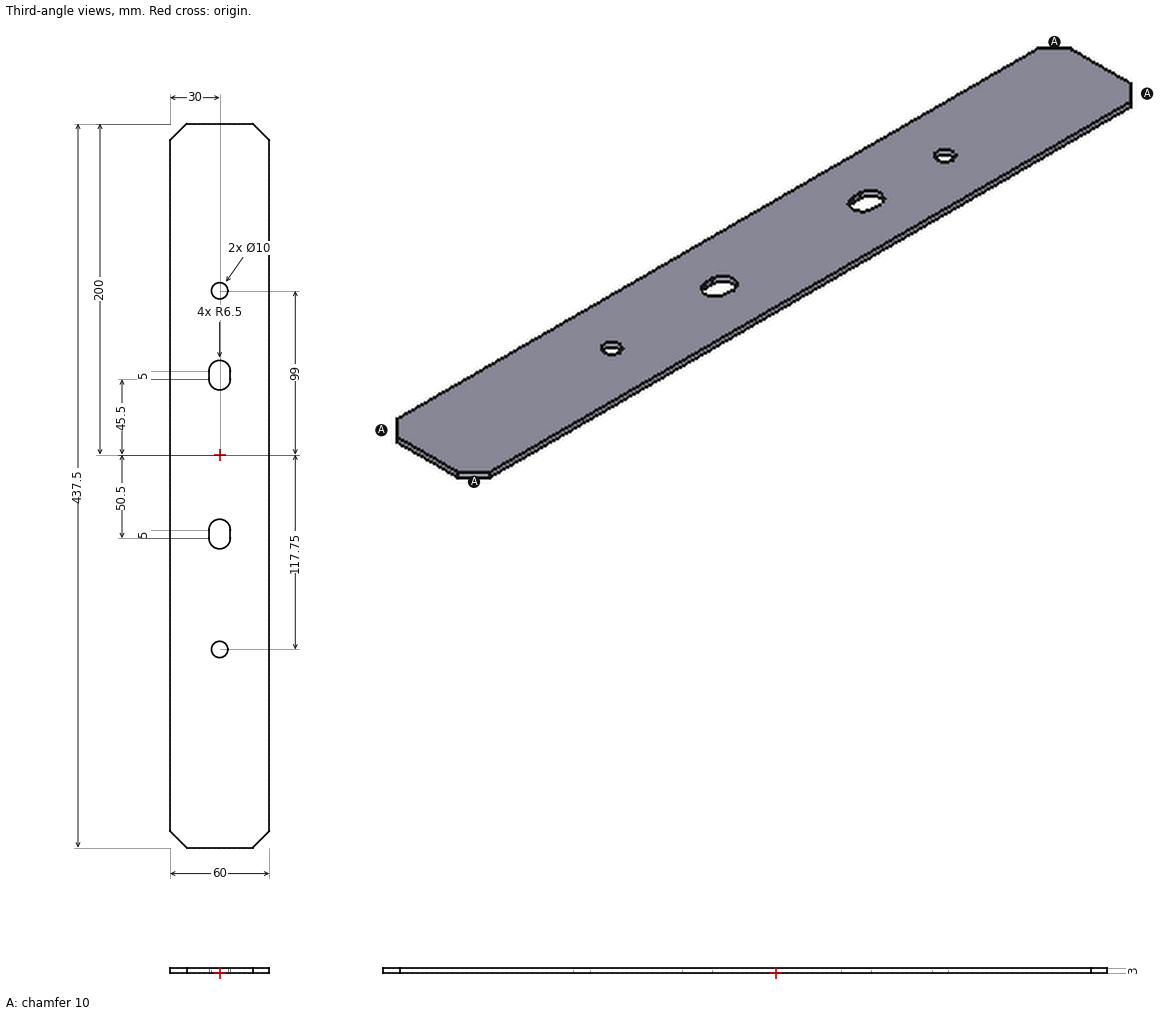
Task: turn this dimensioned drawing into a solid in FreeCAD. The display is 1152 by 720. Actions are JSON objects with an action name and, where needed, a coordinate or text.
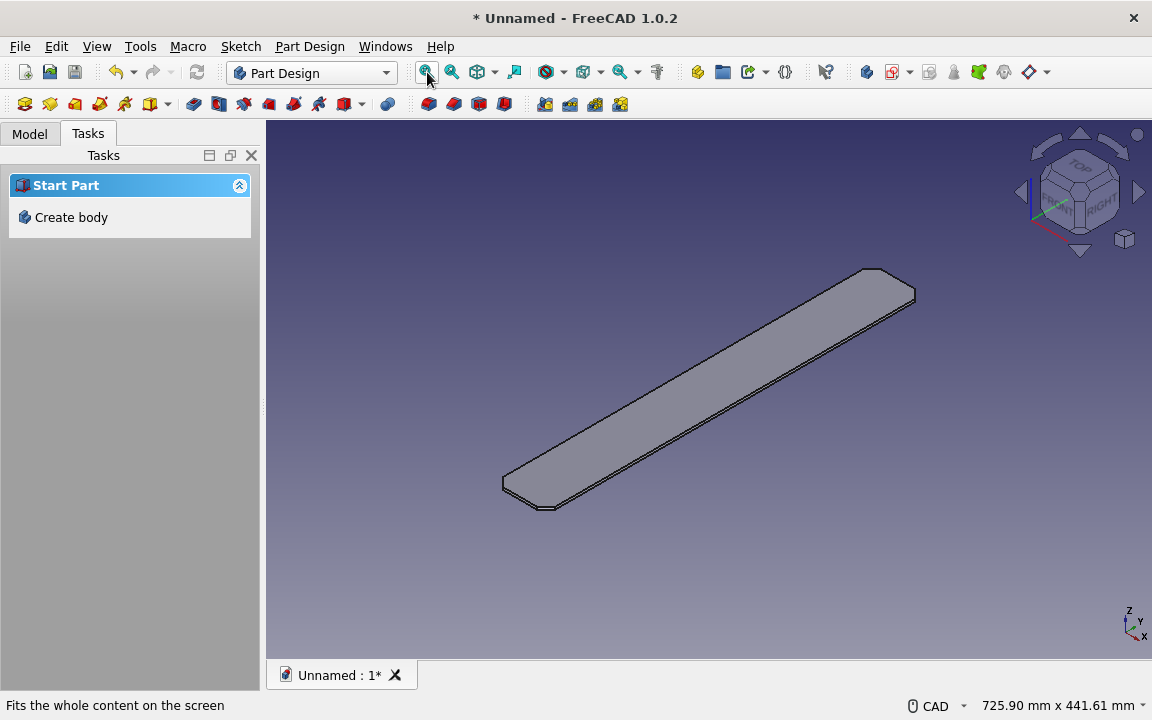
{"action": "left_click", "coordinate": [871, 294]}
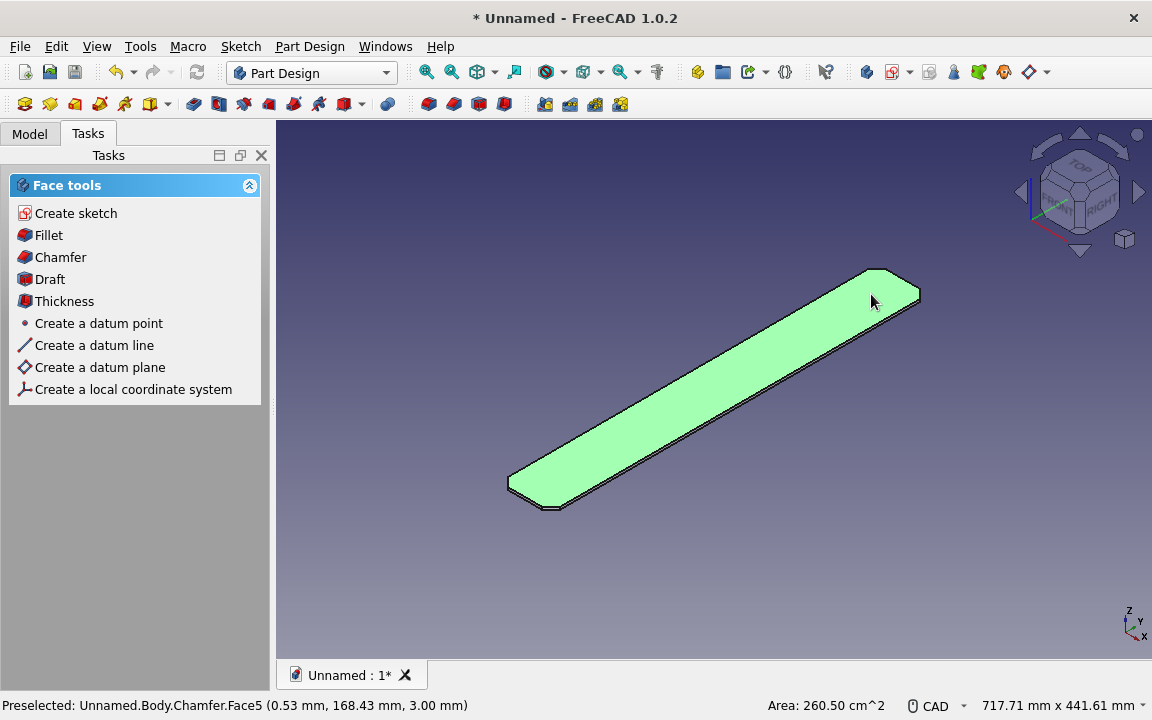
{"action": "left_click", "coordinate": [892, 72]}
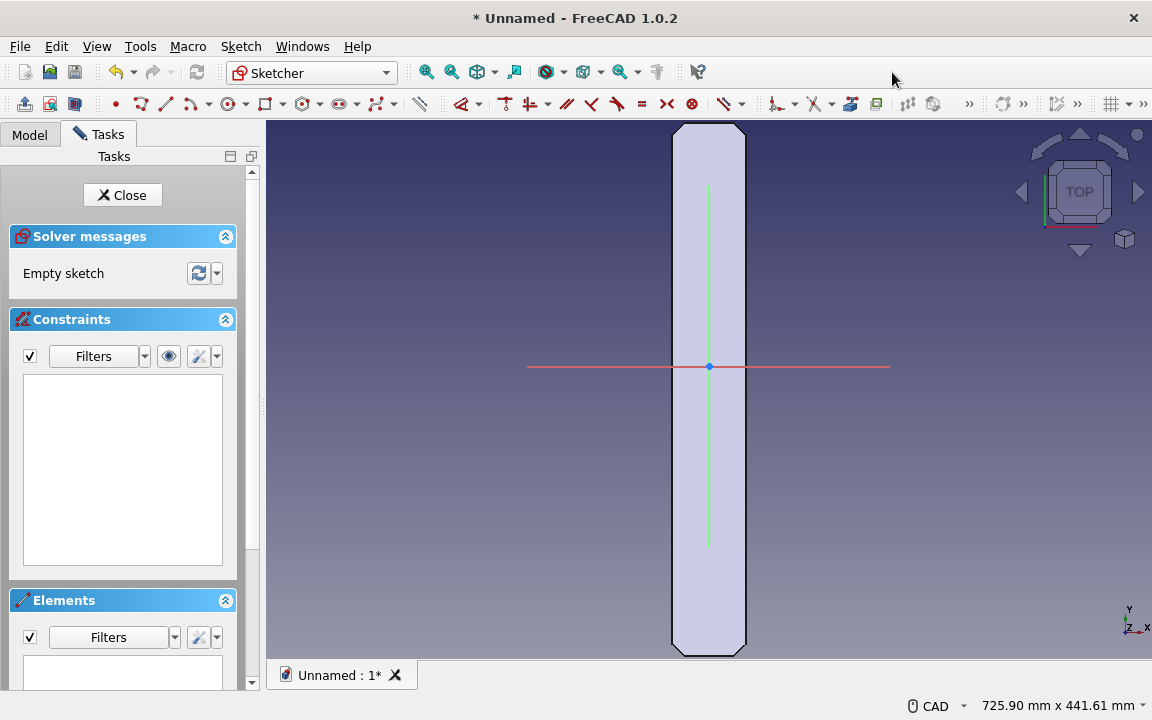
{"action": "left_click", "coordinate": [338, 104]}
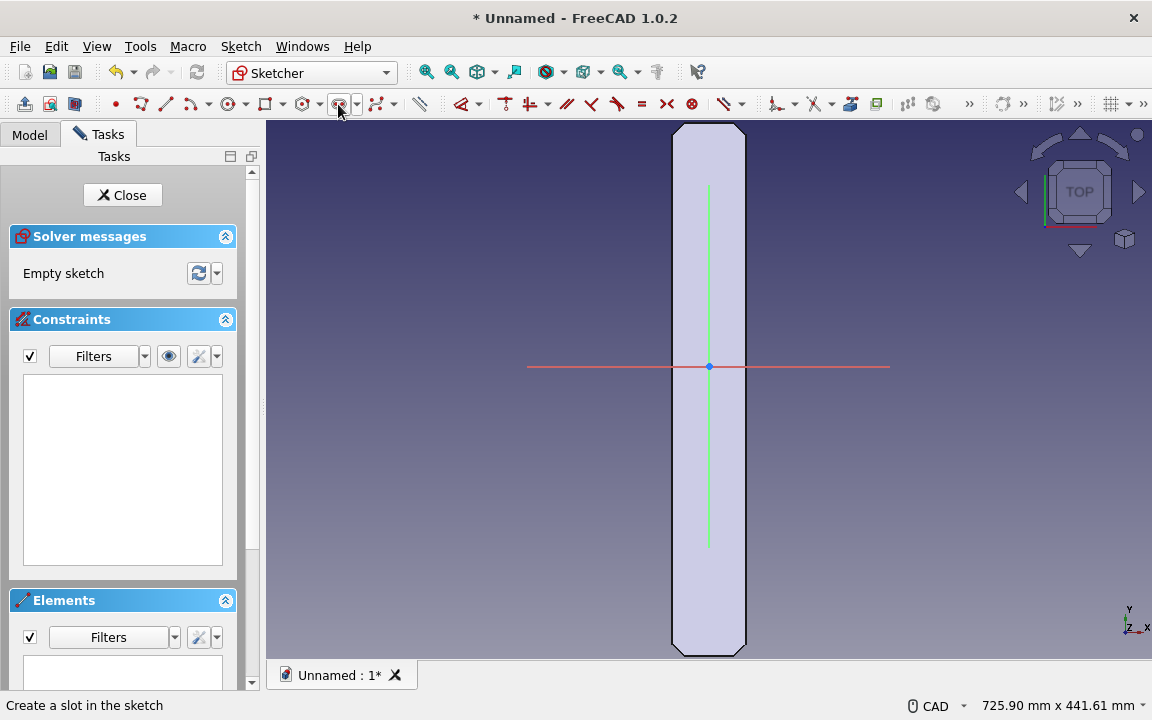
{"action": "scroll", "coordinate": [709, 311], "scroll_direction": "up", "scroll_amount": 6}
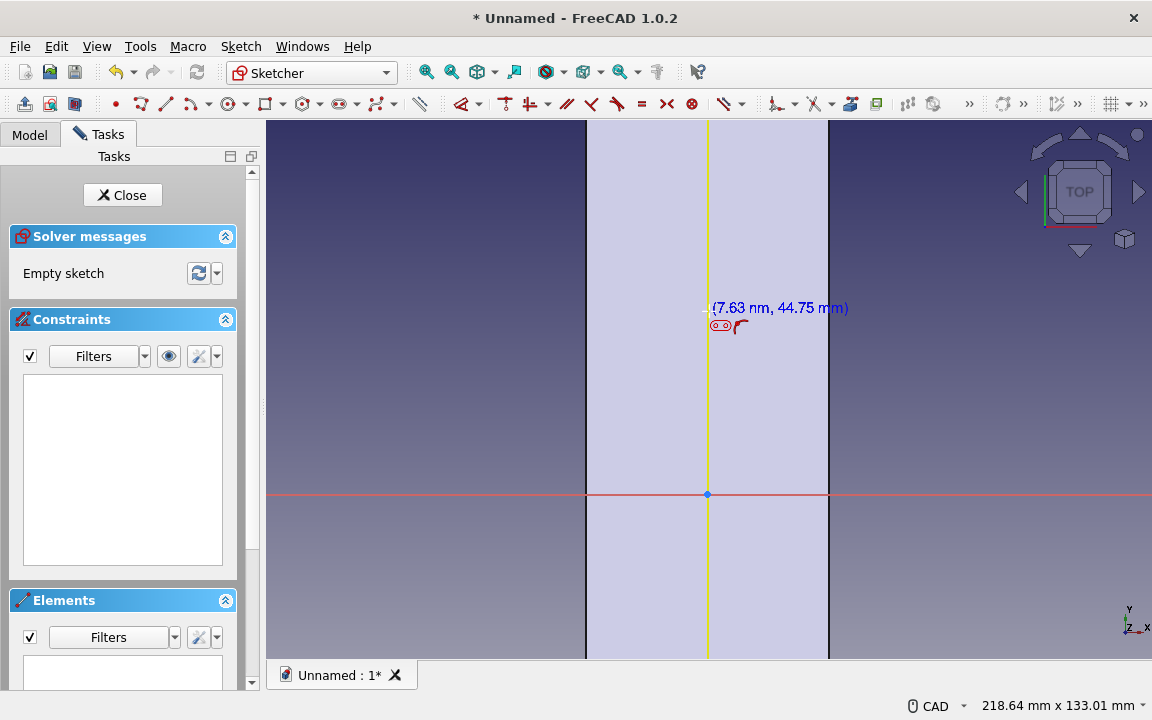
{"action": "left_click", "coordinate": [708, 310]}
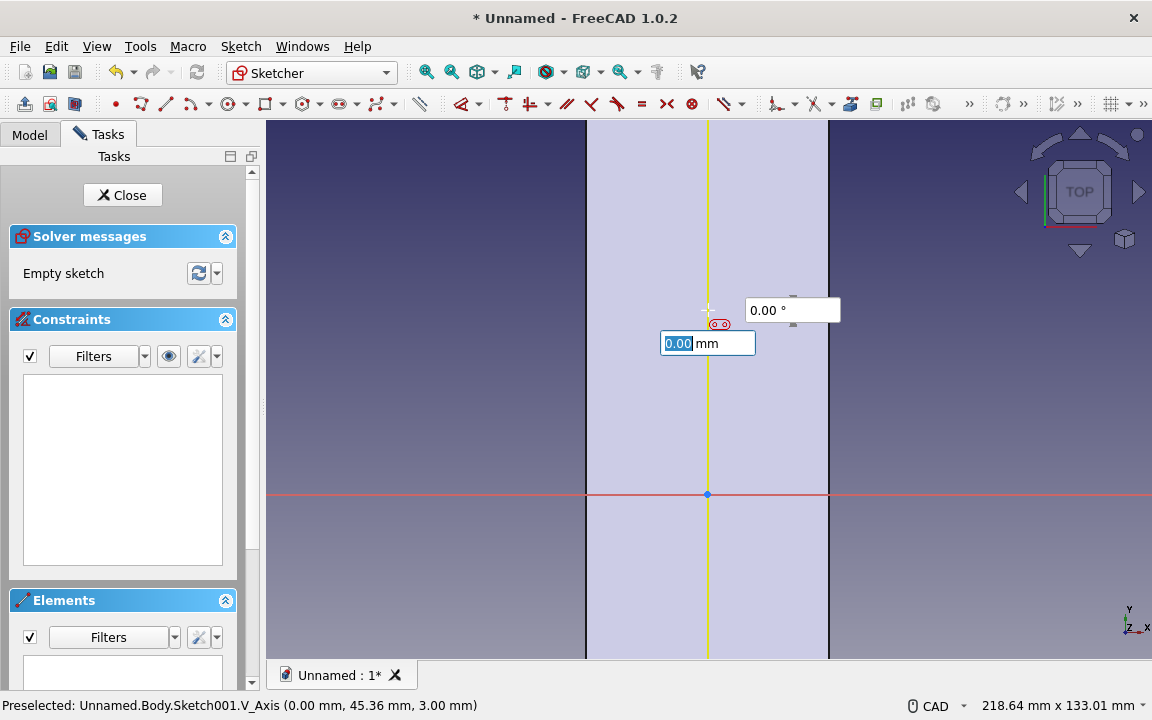
{"action": "left_click", "coordinate": [717, 290]}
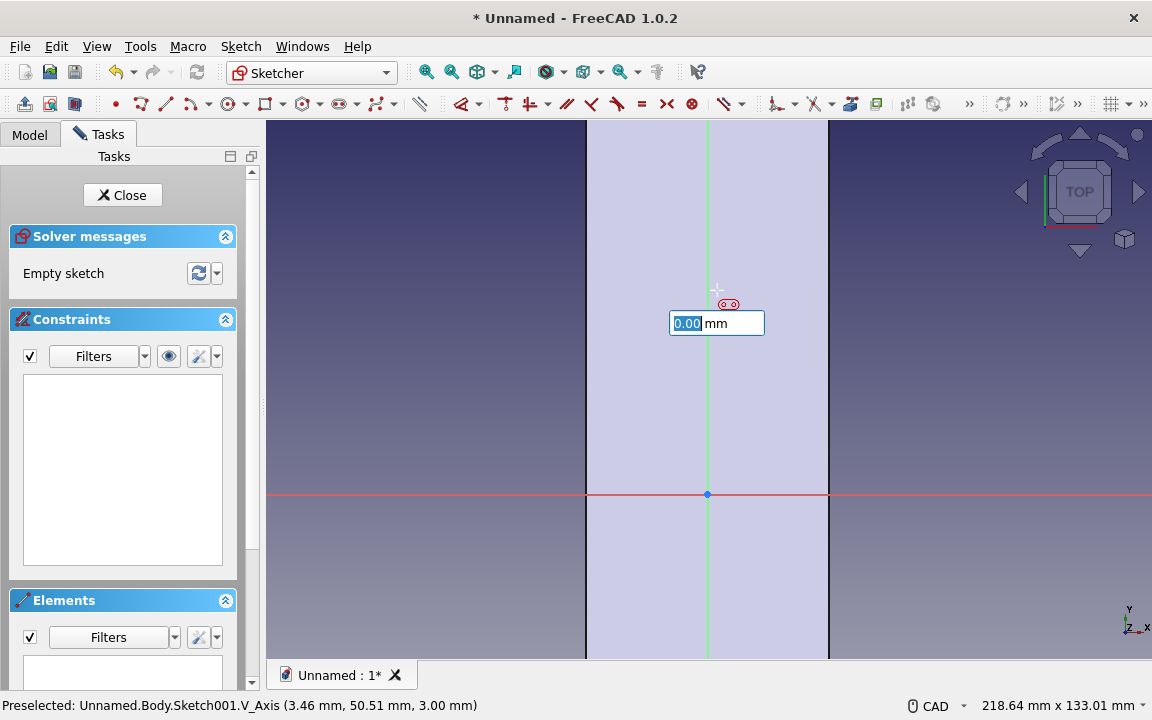
{"action": "left_click", "coordinate": [734, 300]}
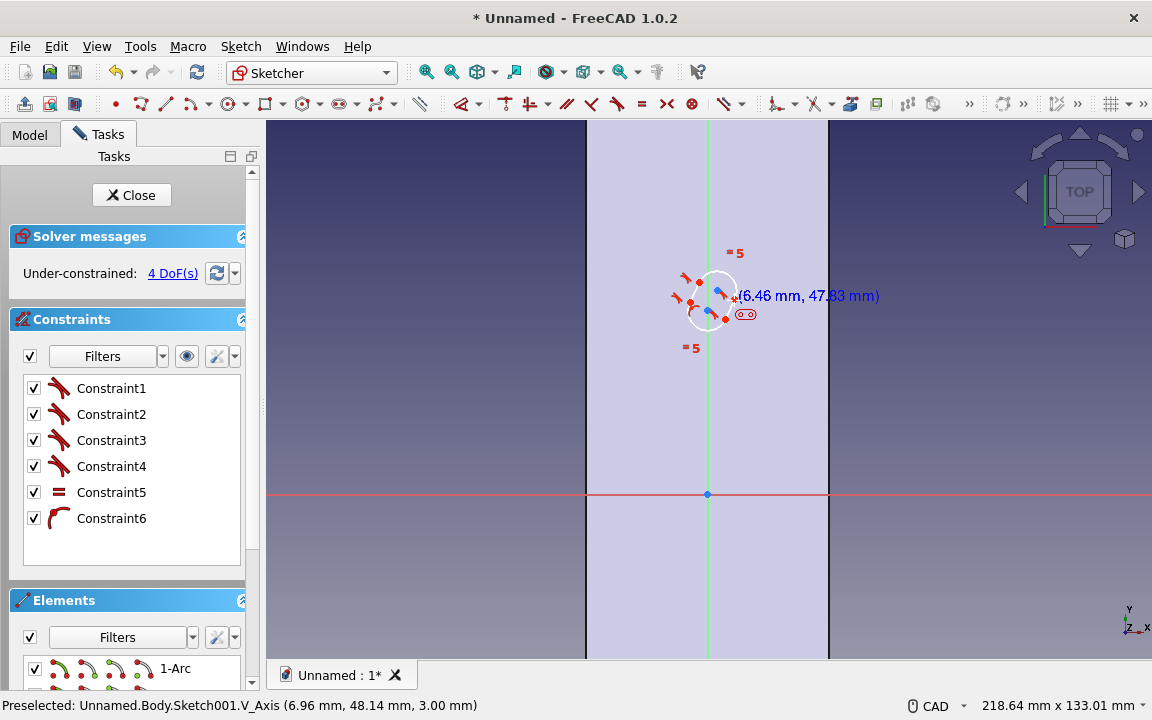
{"action": "scroll", "coordinate": [601, 306], "scroll_direction": "down", "scroll_amount": 5}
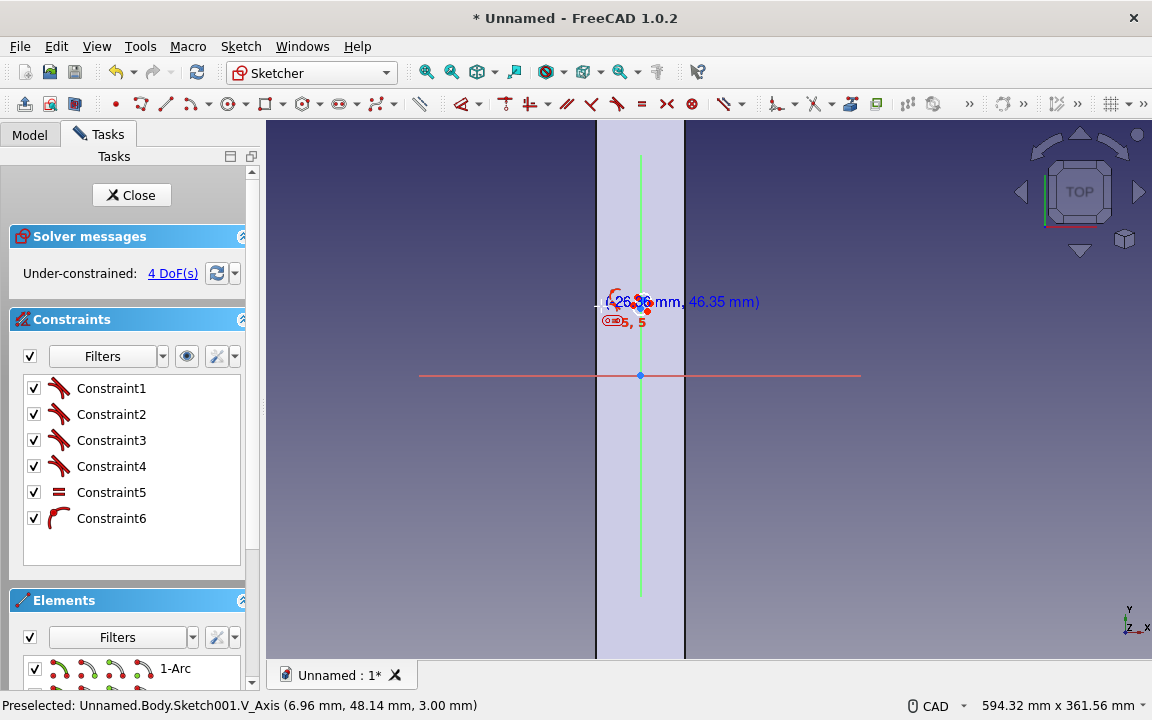
{"action": "scroll", "coordinate": [641, 451], "scroll_direction": "up", "scroll_amount": 5}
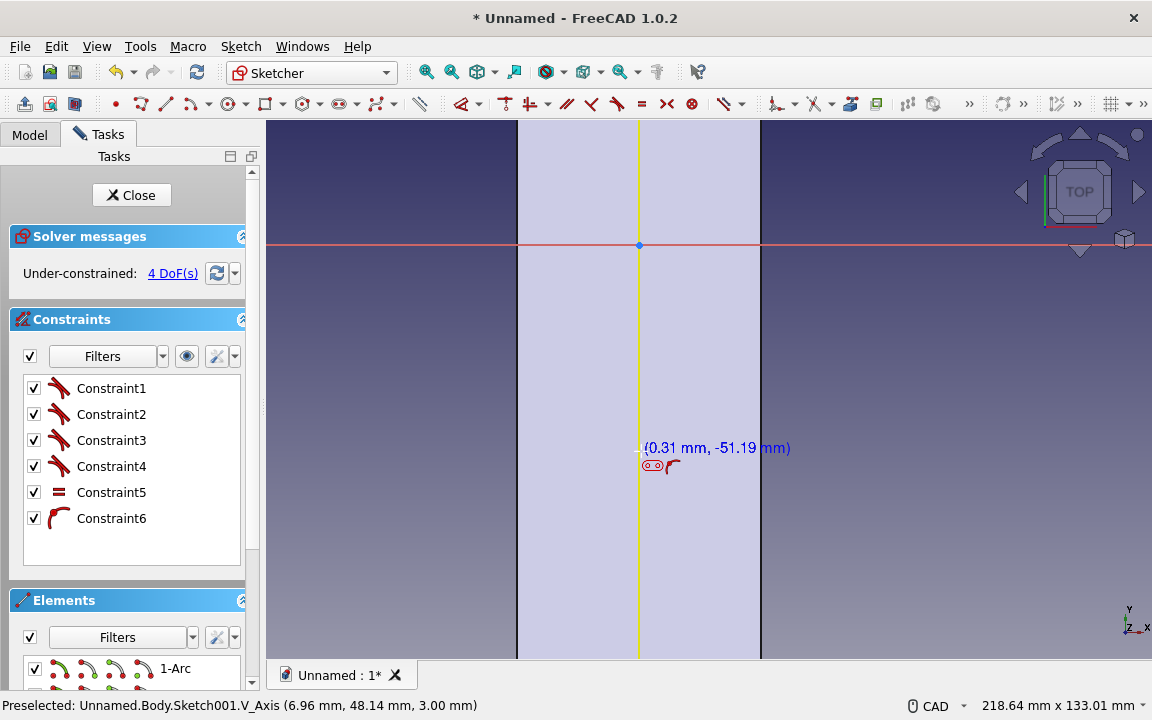
{"action": "left_click", "coordinate": [639, 450]}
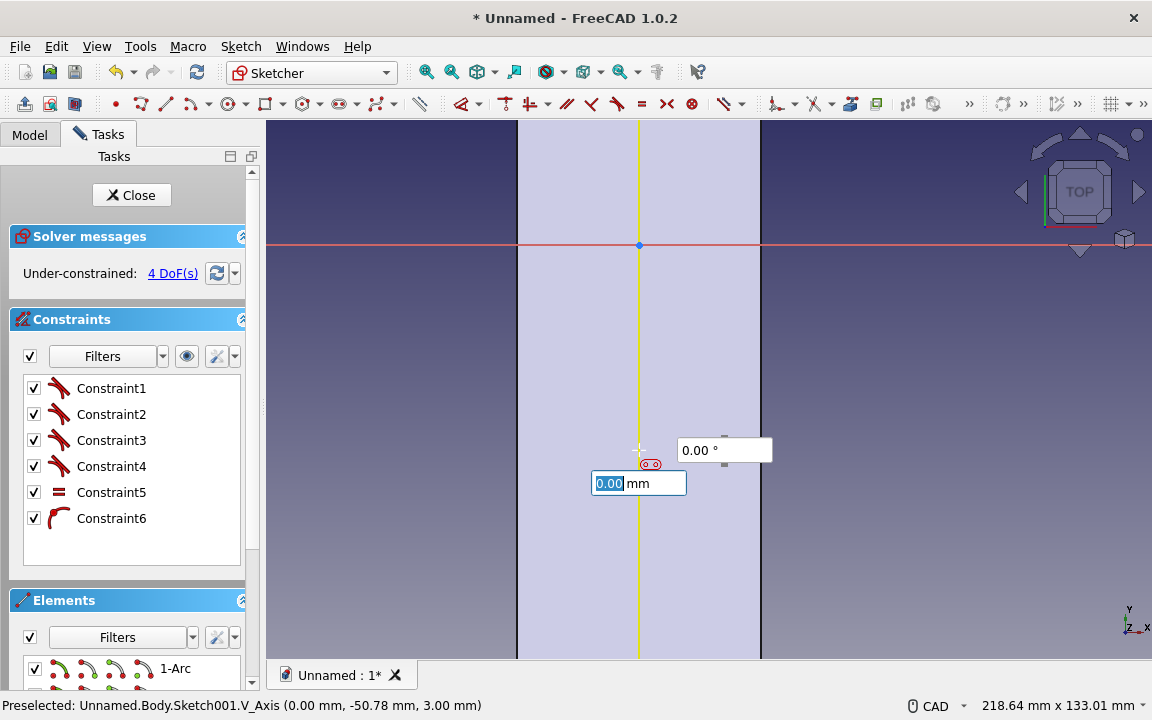
{"action": "left_click", "coordinate": [648, 430]}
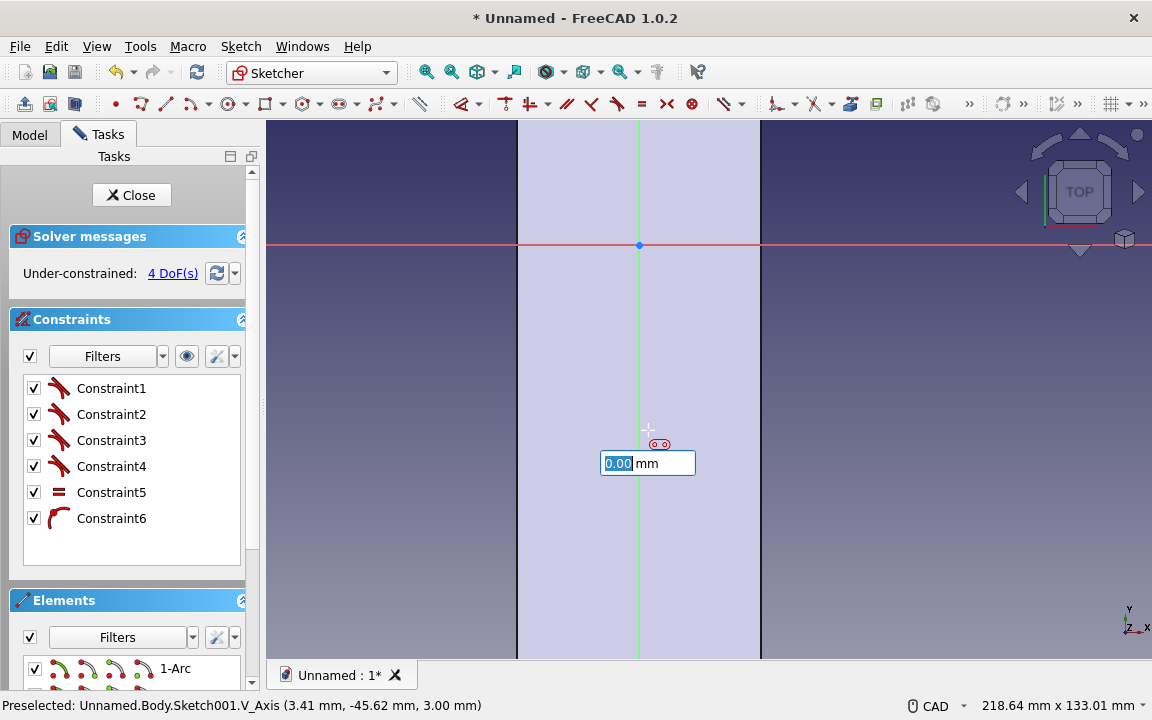
{"action": "left_click", "coordinate": [665, 440]}